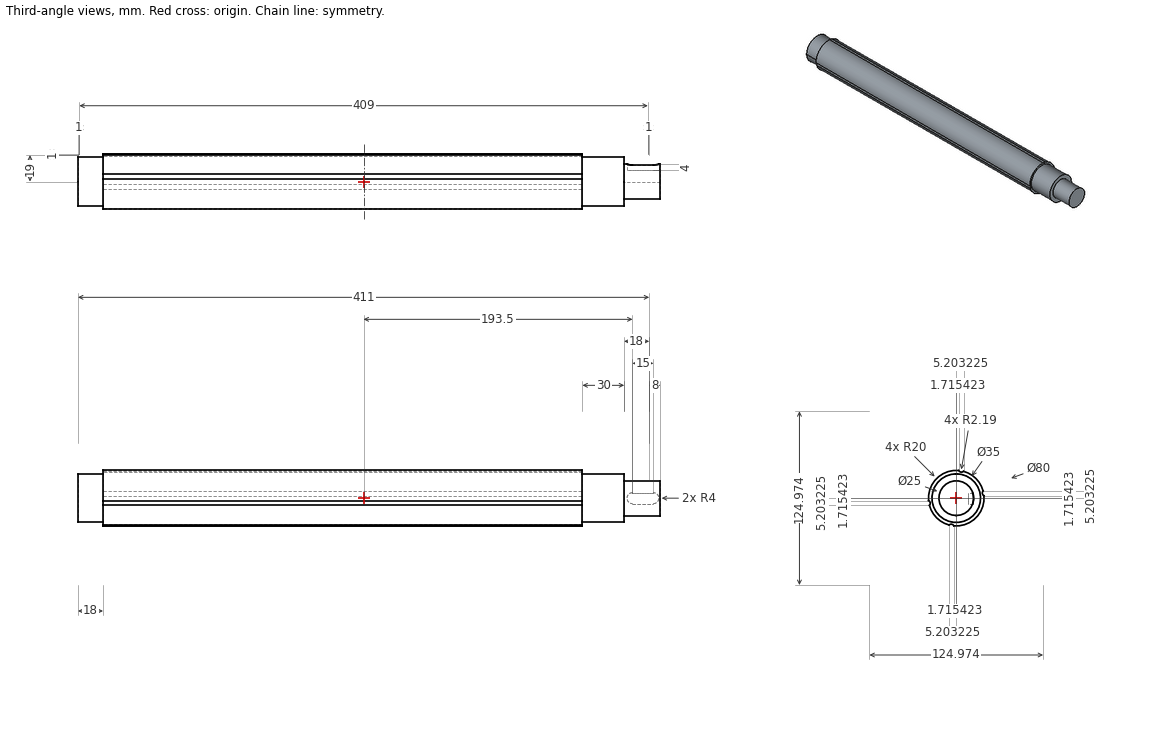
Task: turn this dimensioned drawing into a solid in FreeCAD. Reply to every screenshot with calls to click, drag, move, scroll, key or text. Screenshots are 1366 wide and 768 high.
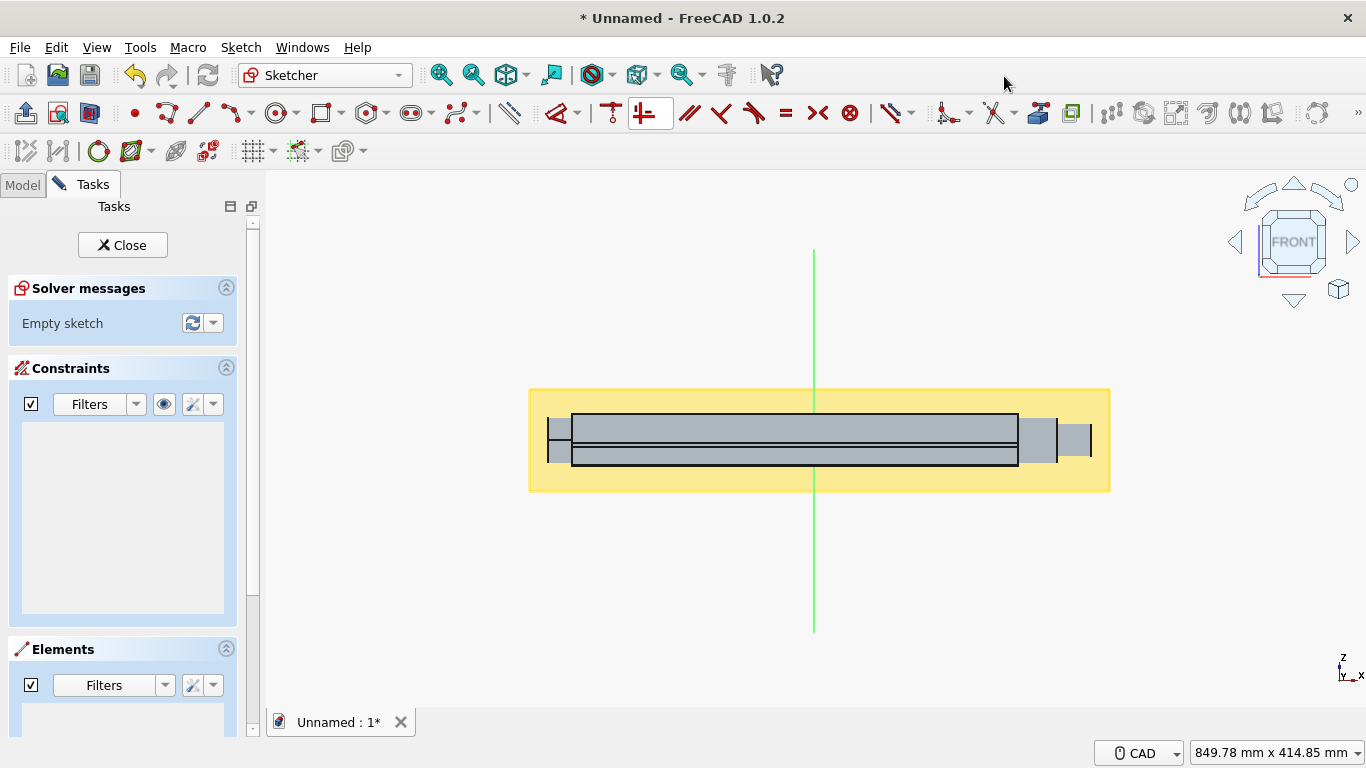
click(90, 114)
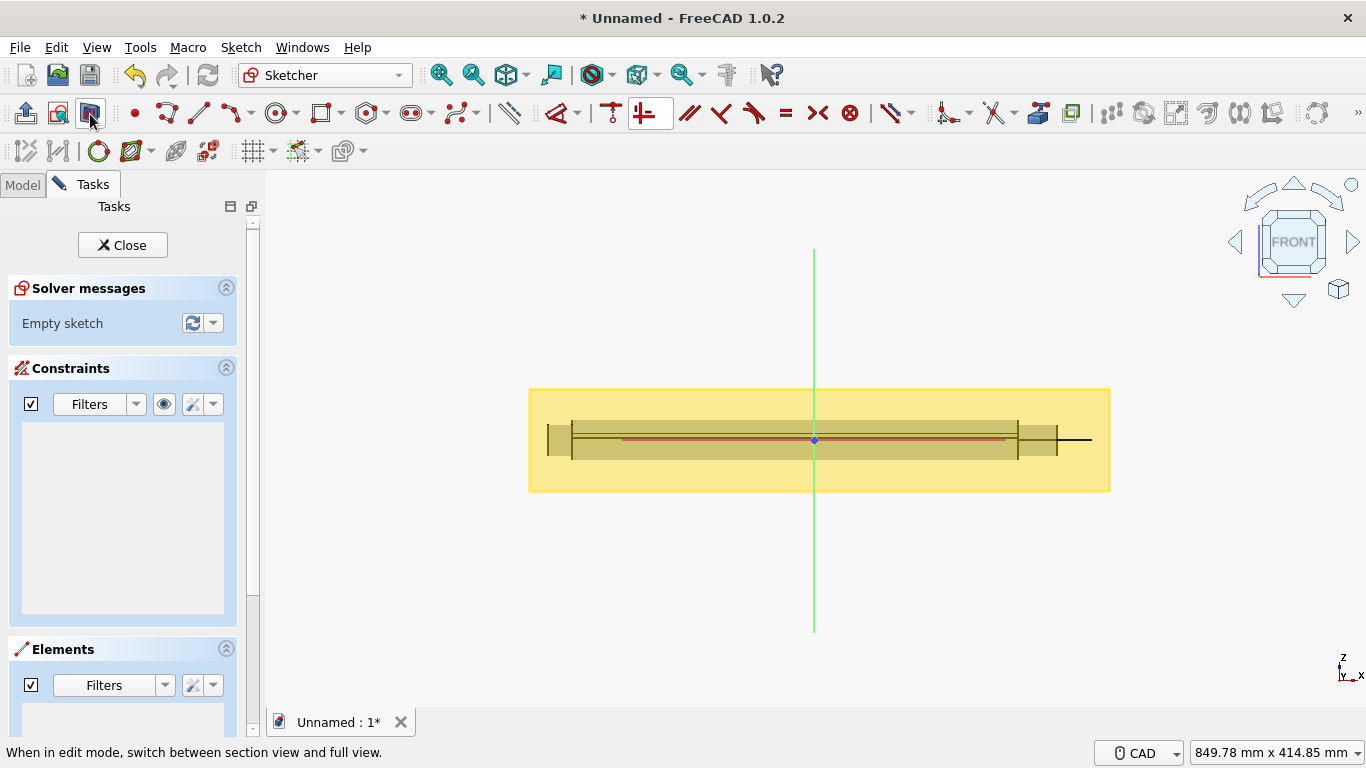
scroll(1092, 440, up, 15)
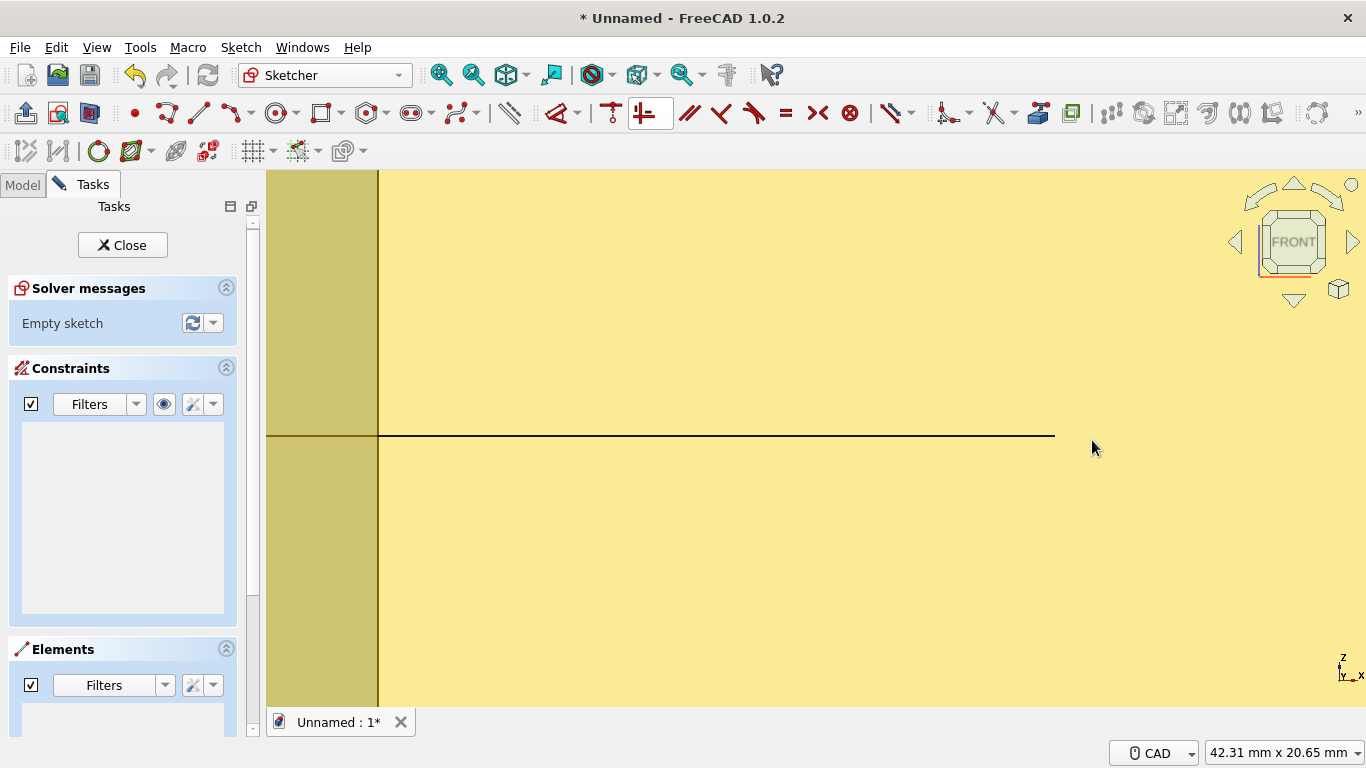
key(g)
key(s)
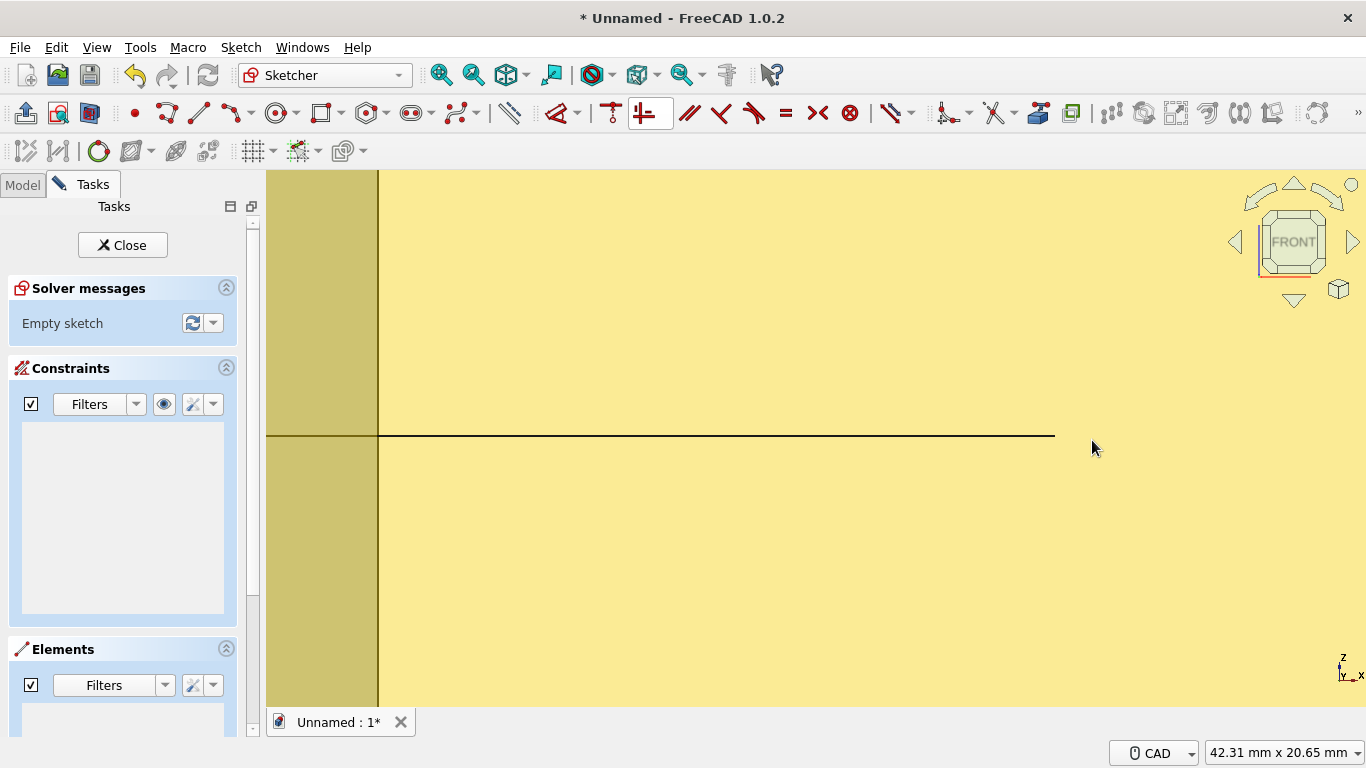
click(534, 436)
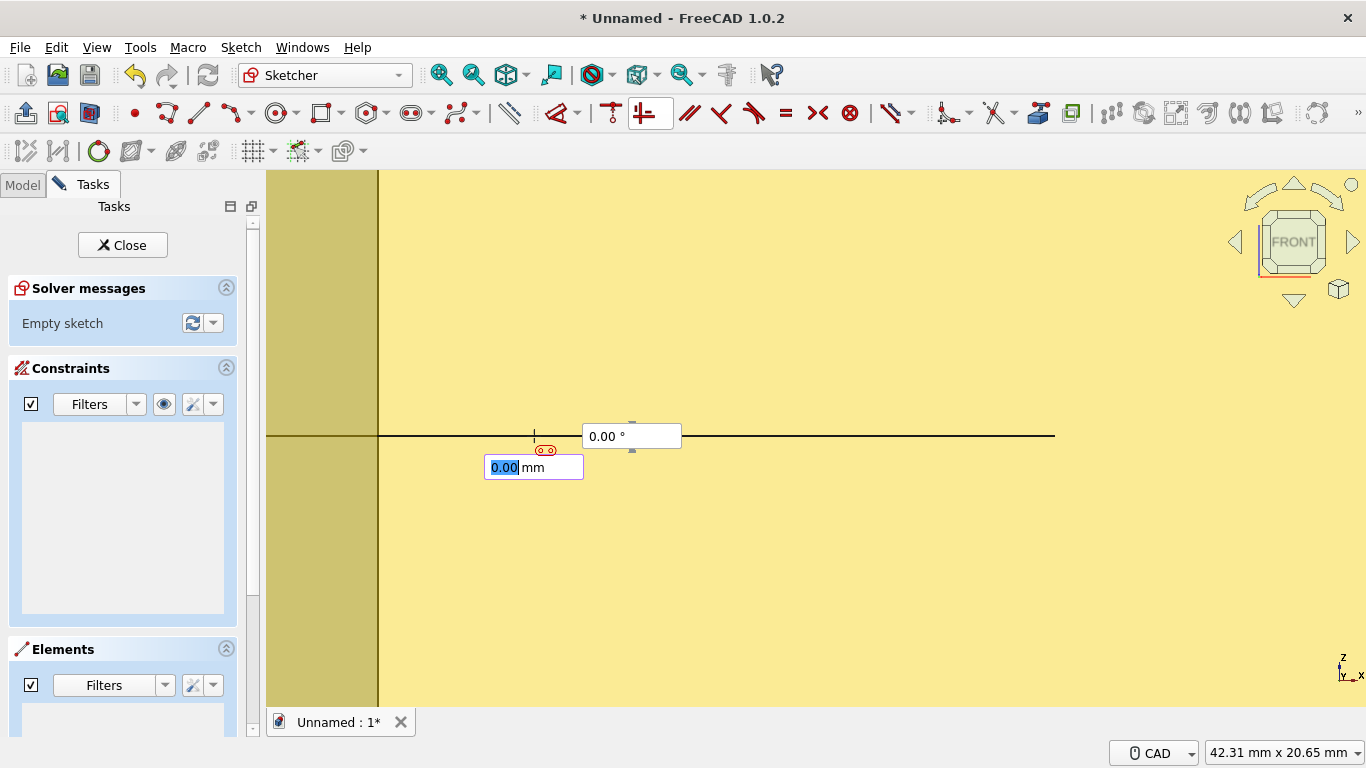
click(924, 427)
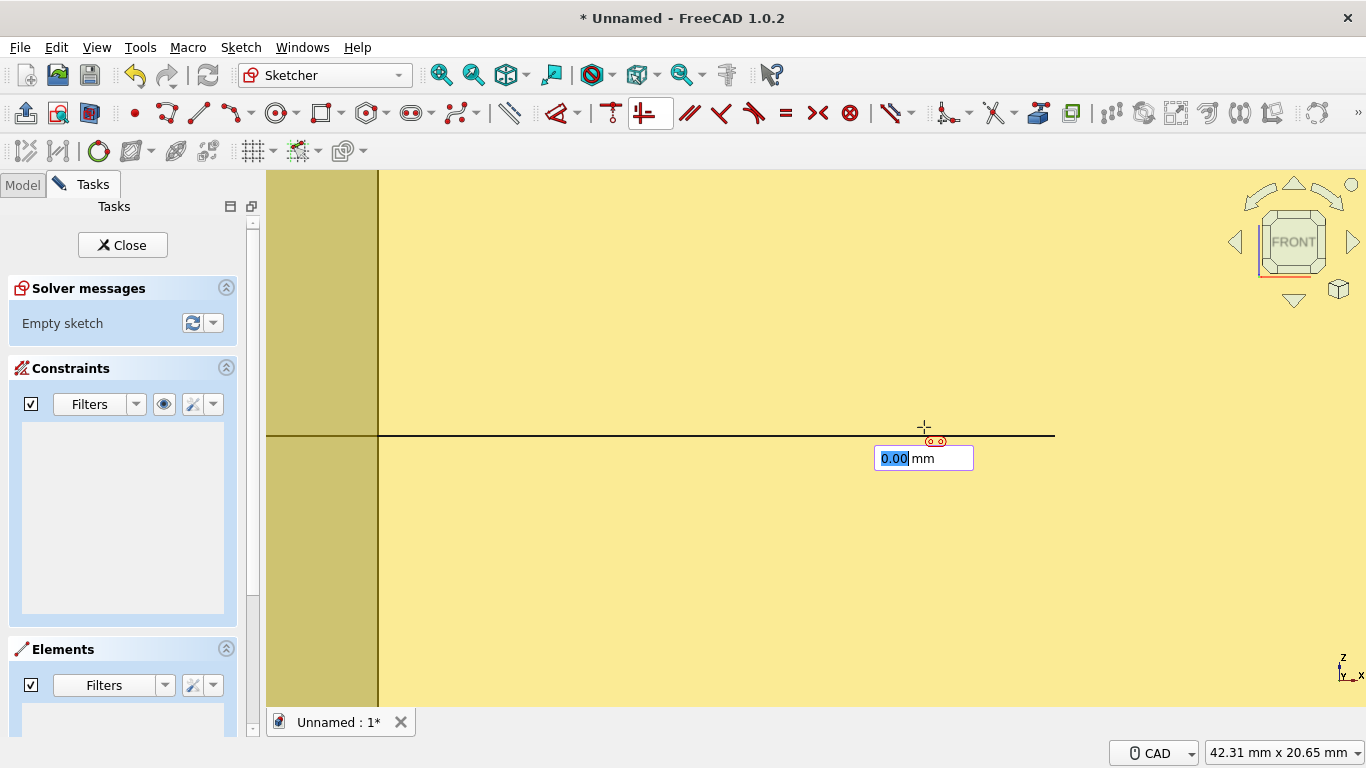
click(729, 332)
key(Escape)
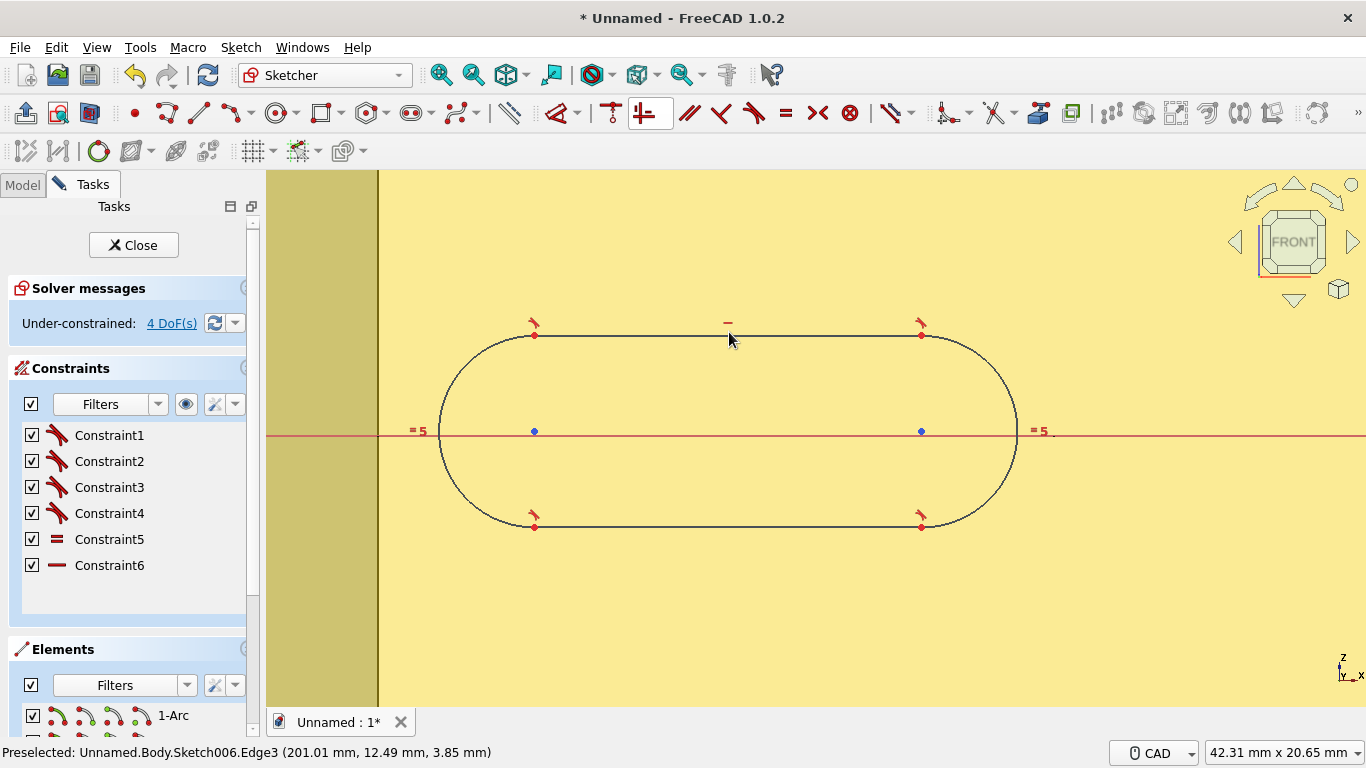
click(535, 432)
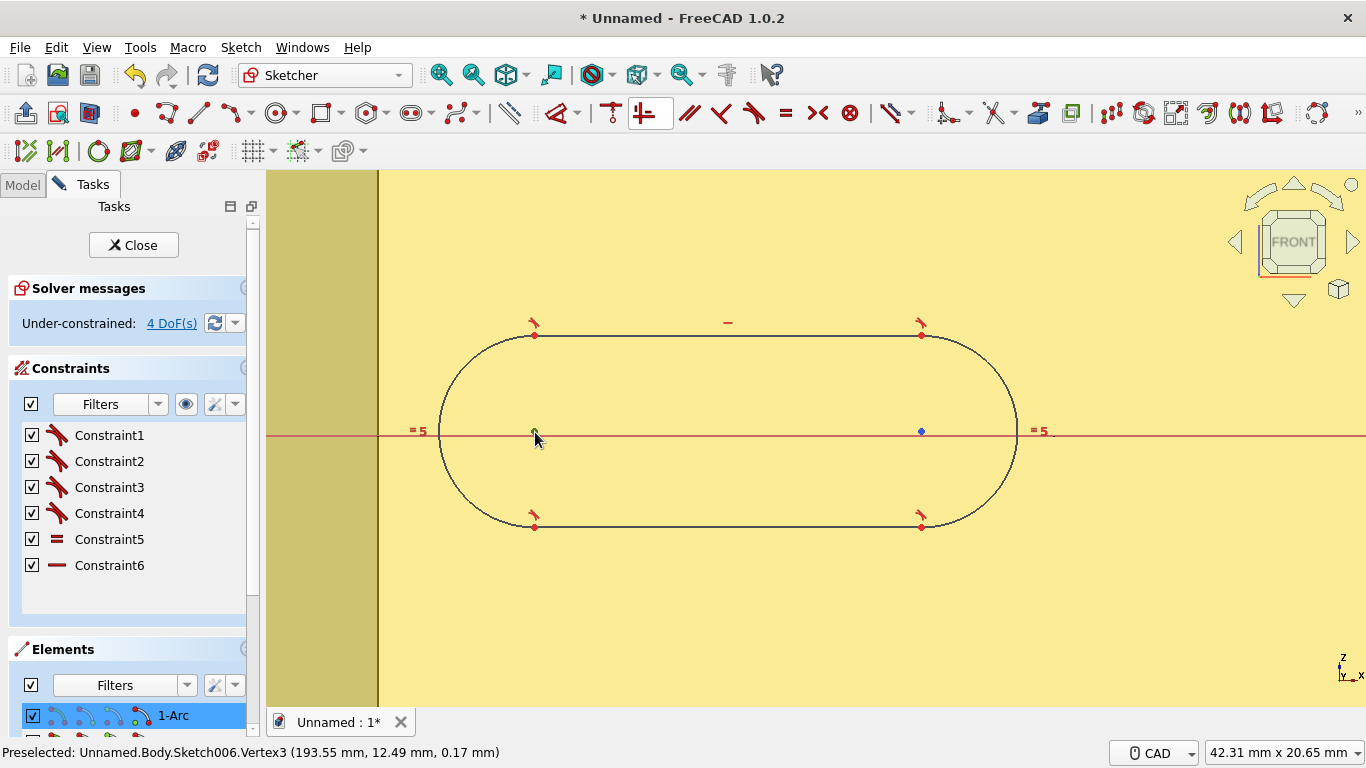
click(359, 436)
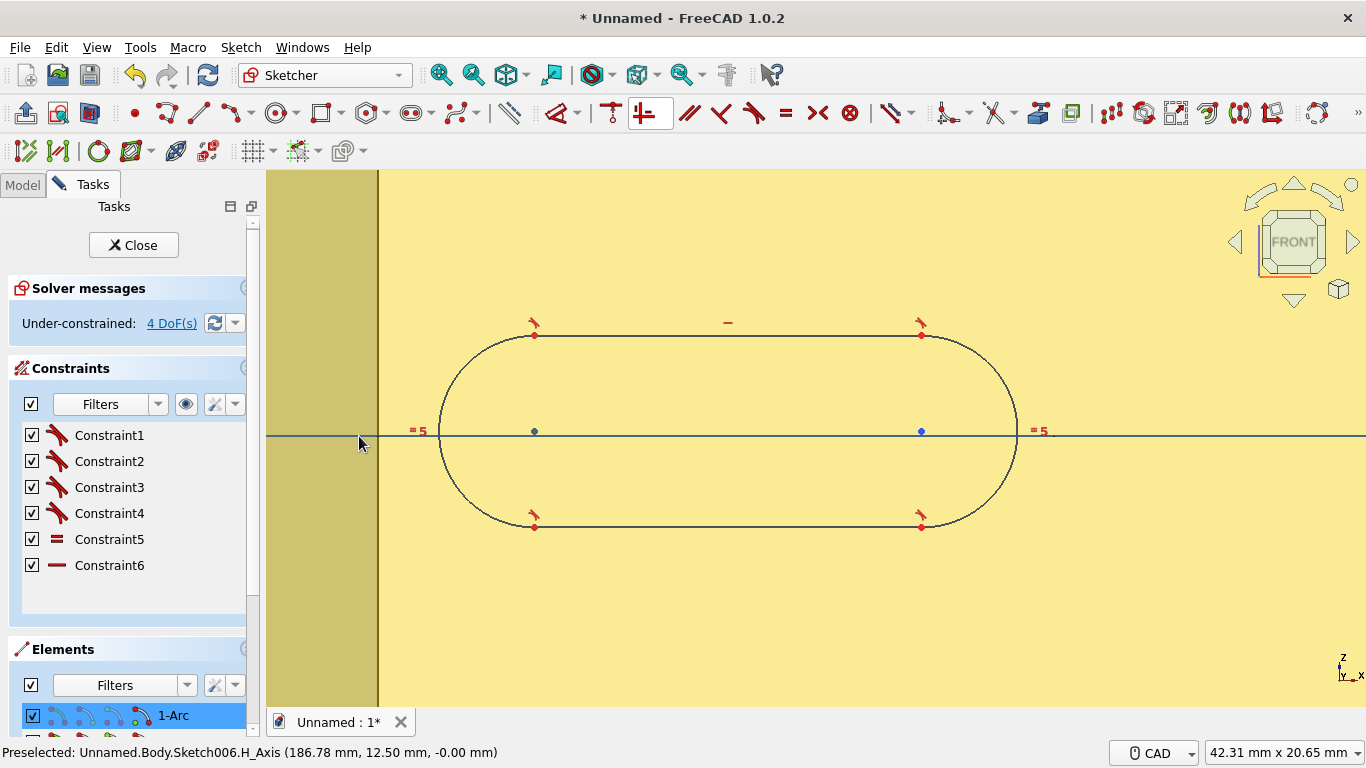
click(612, 114)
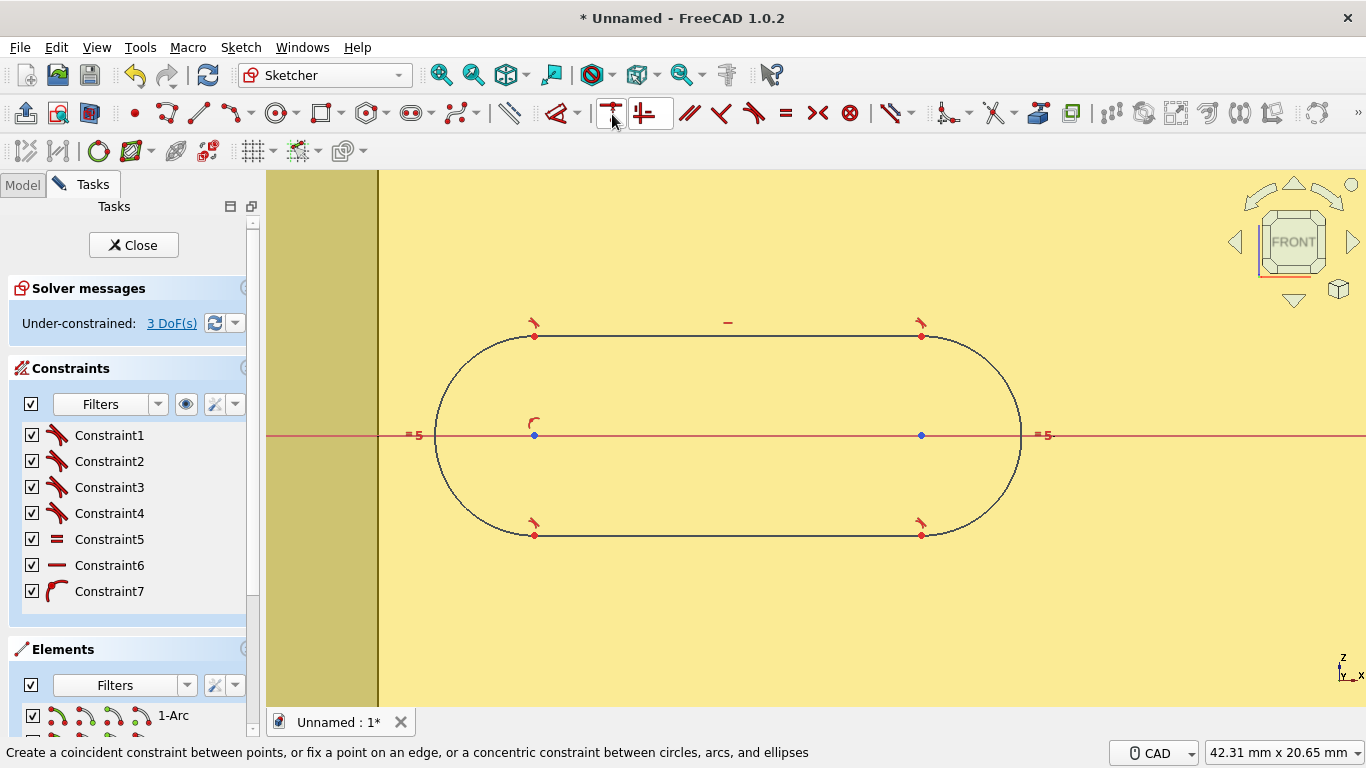
key(d)